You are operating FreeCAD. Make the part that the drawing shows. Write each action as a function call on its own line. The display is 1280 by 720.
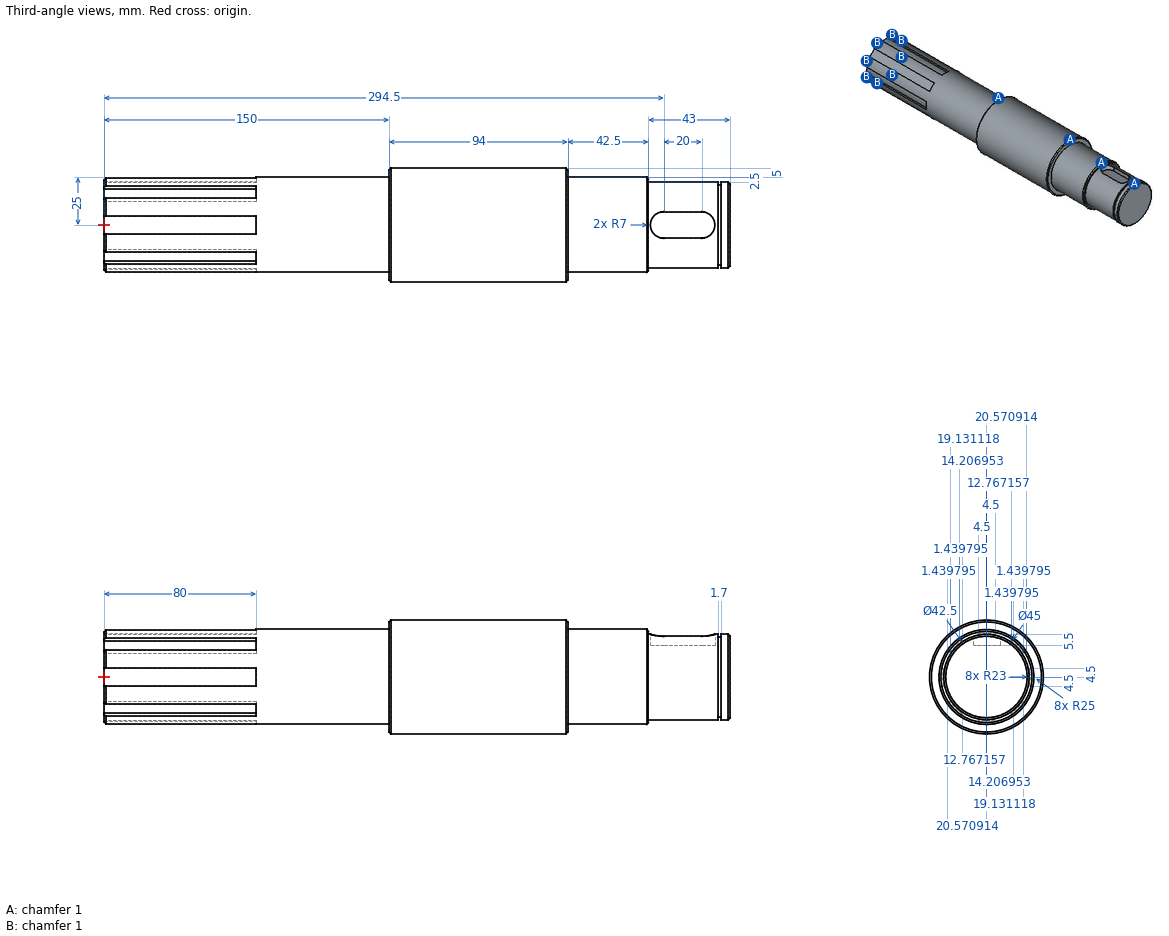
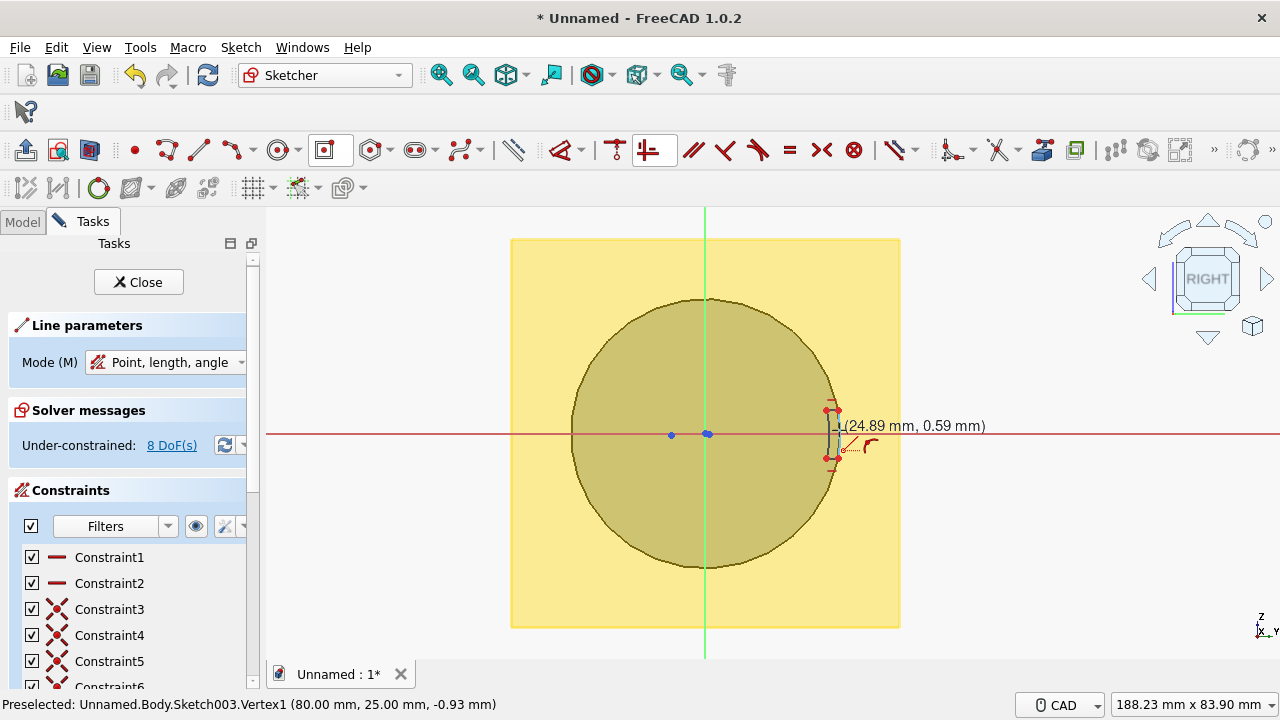
click(774, 331)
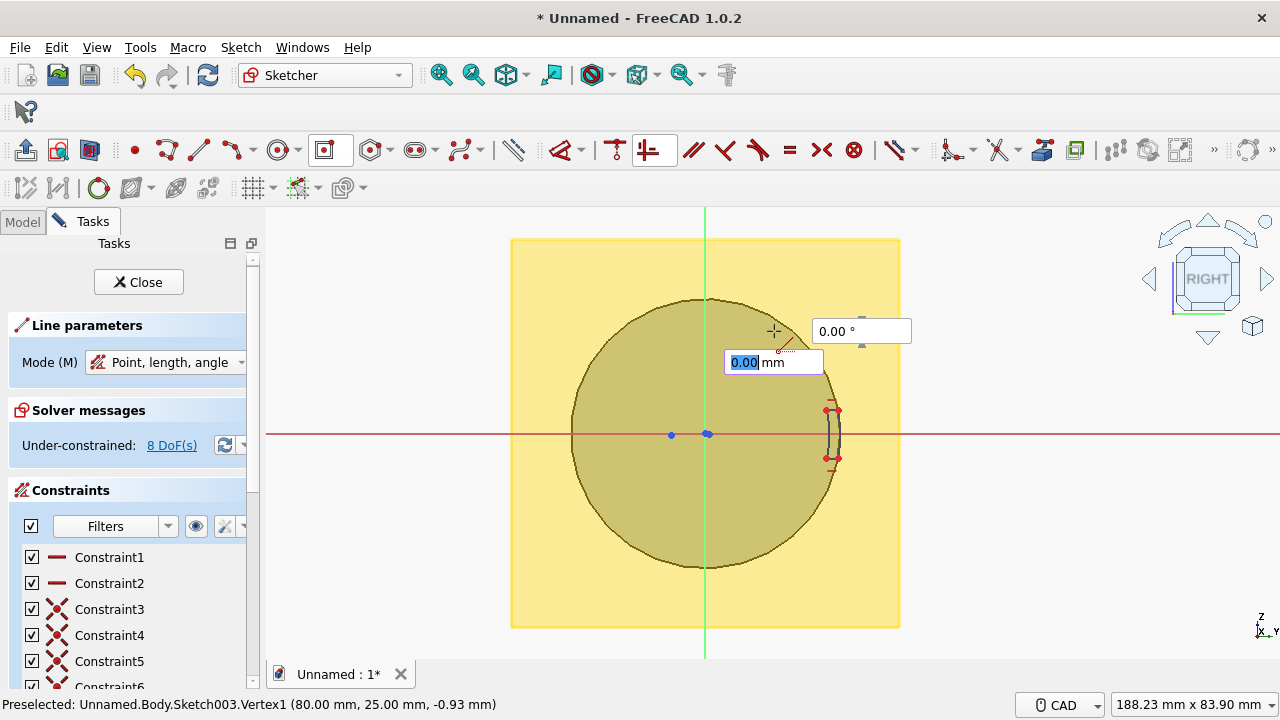
scroll(782, 323, up, 2)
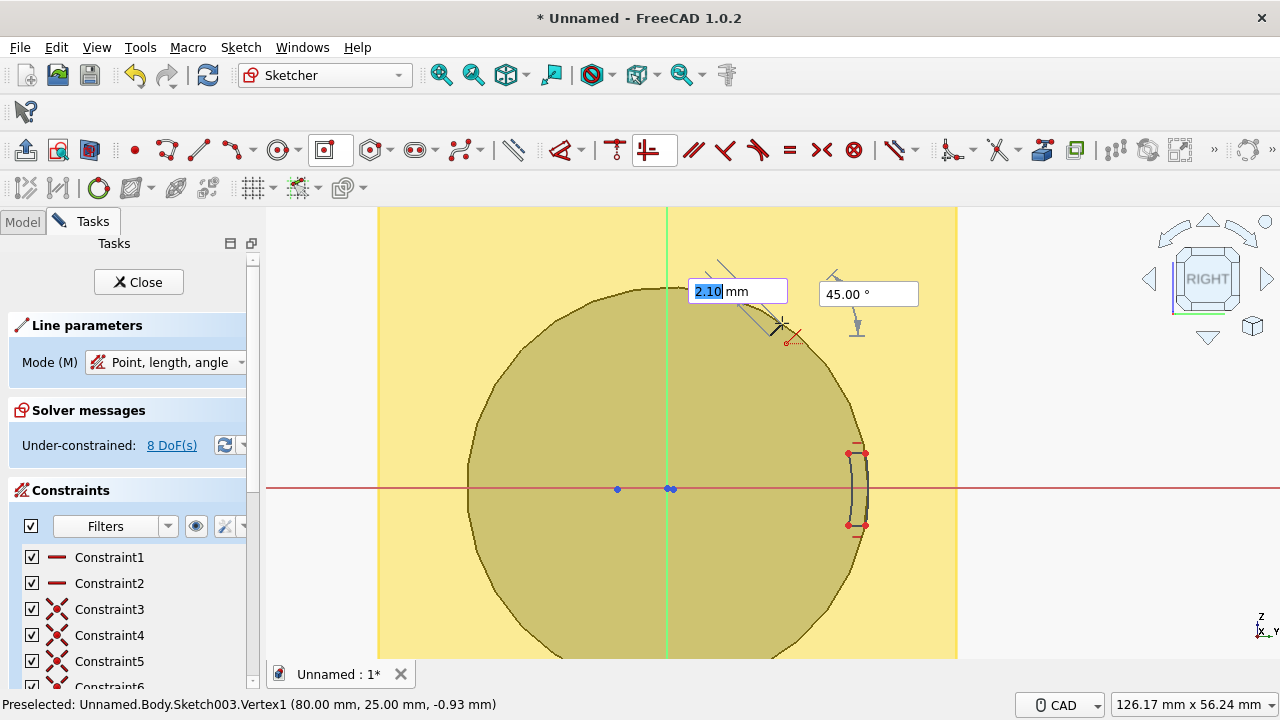
click(782, 323)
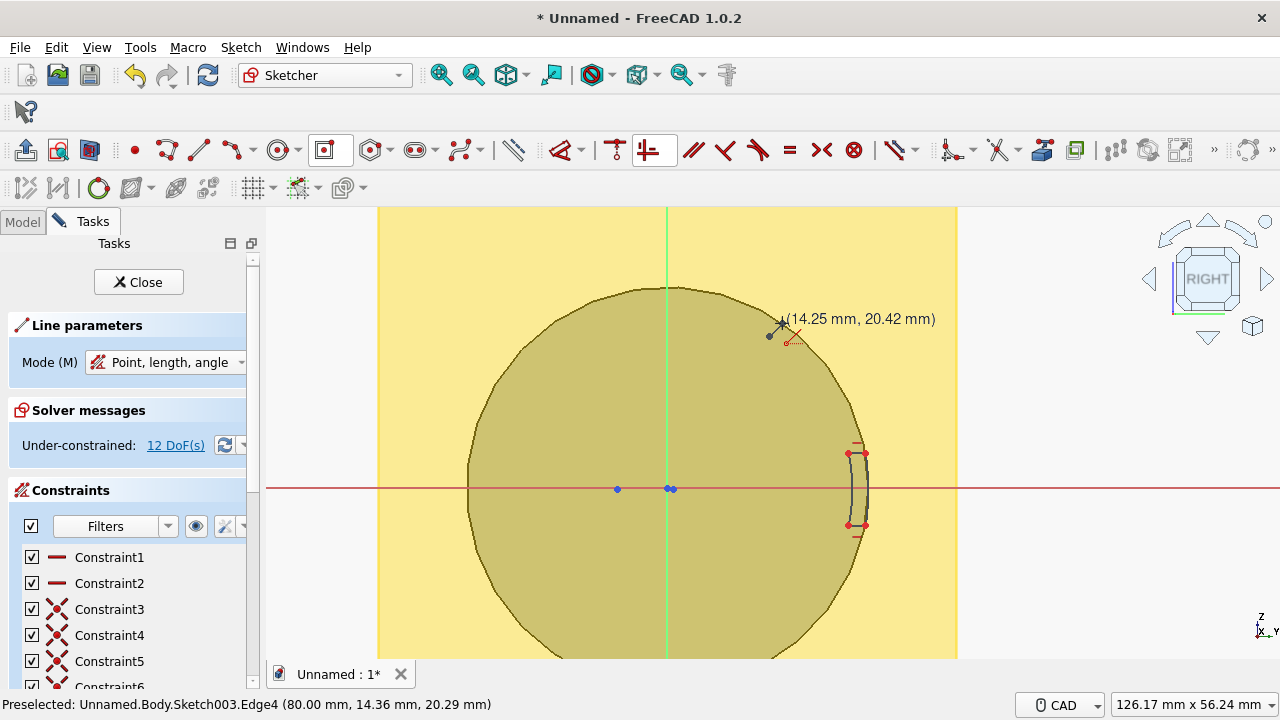
click(833, 374)
click(821, 385)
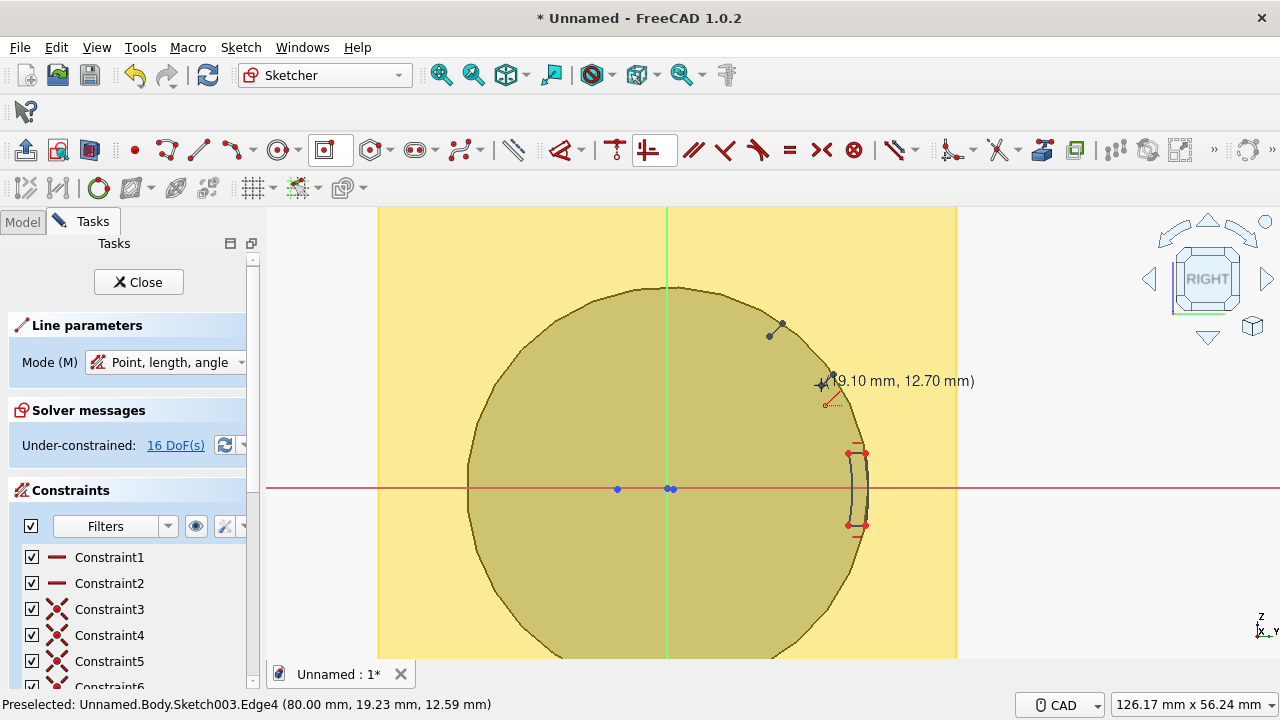
click(232, 150)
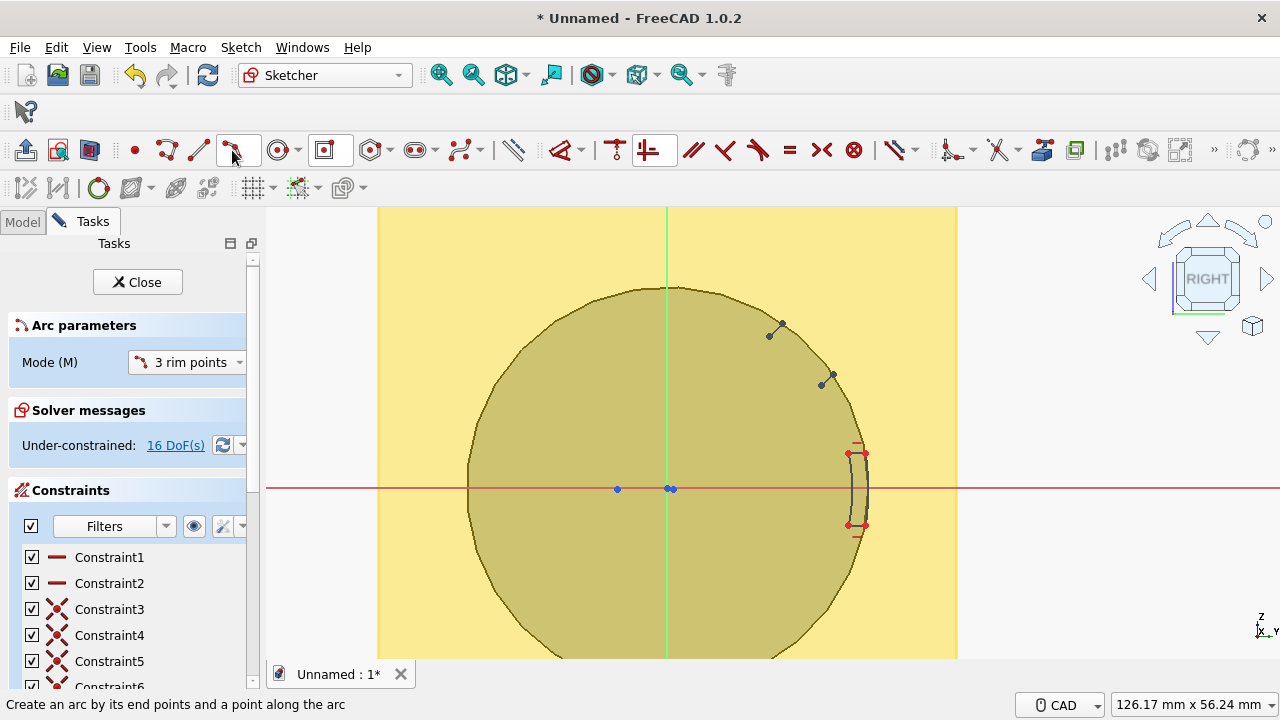
scroll(782, 323, up, 4)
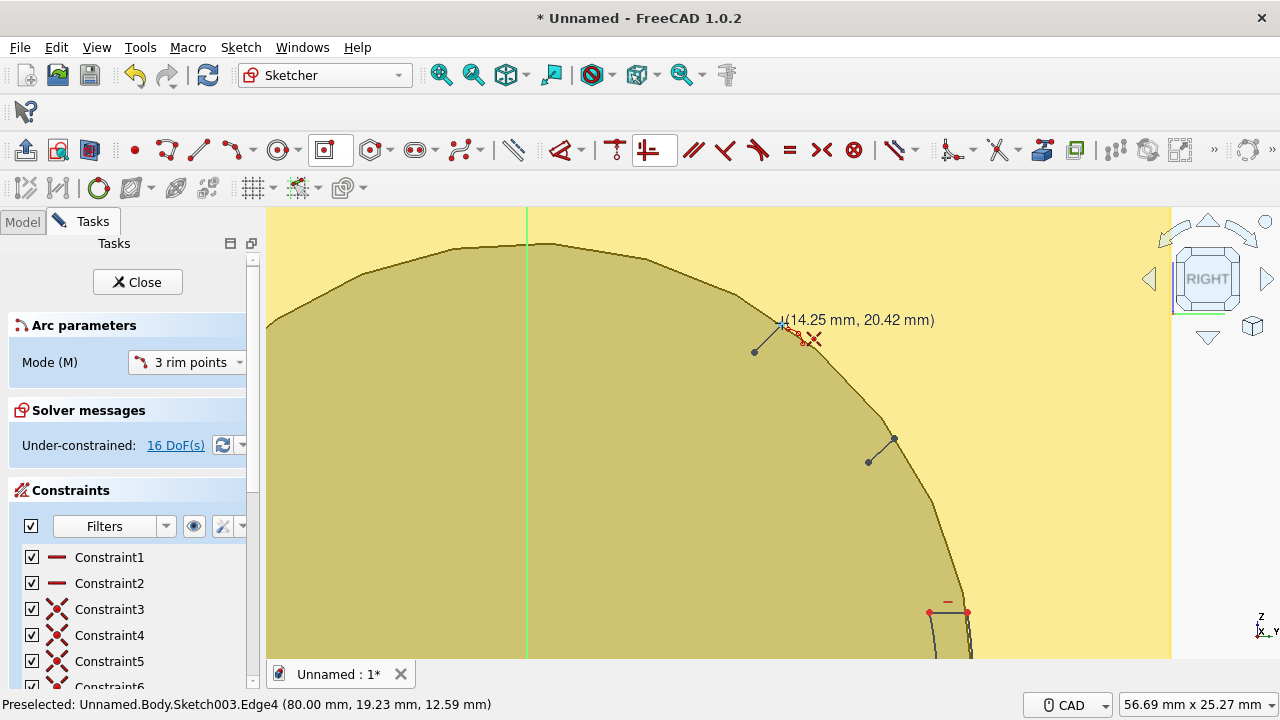
click(781, 325)
click(895, 438)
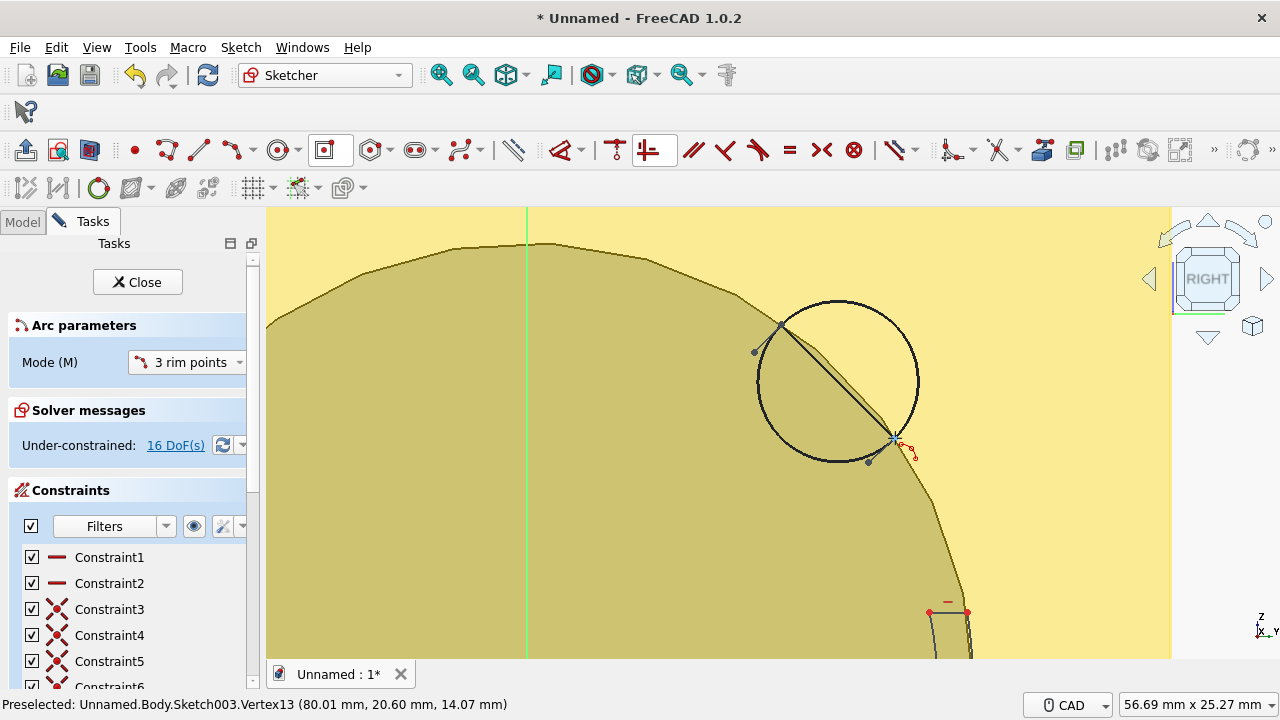
scroll(843, 374, up, 4)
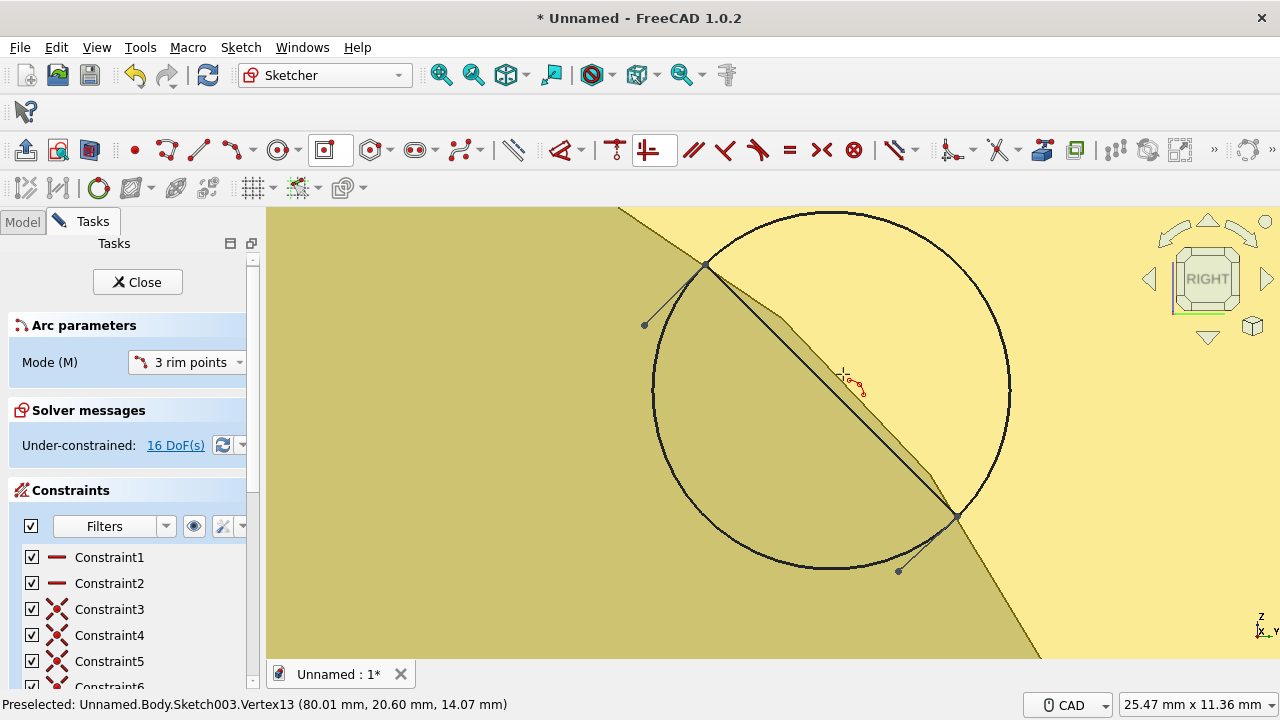
click(842, 373)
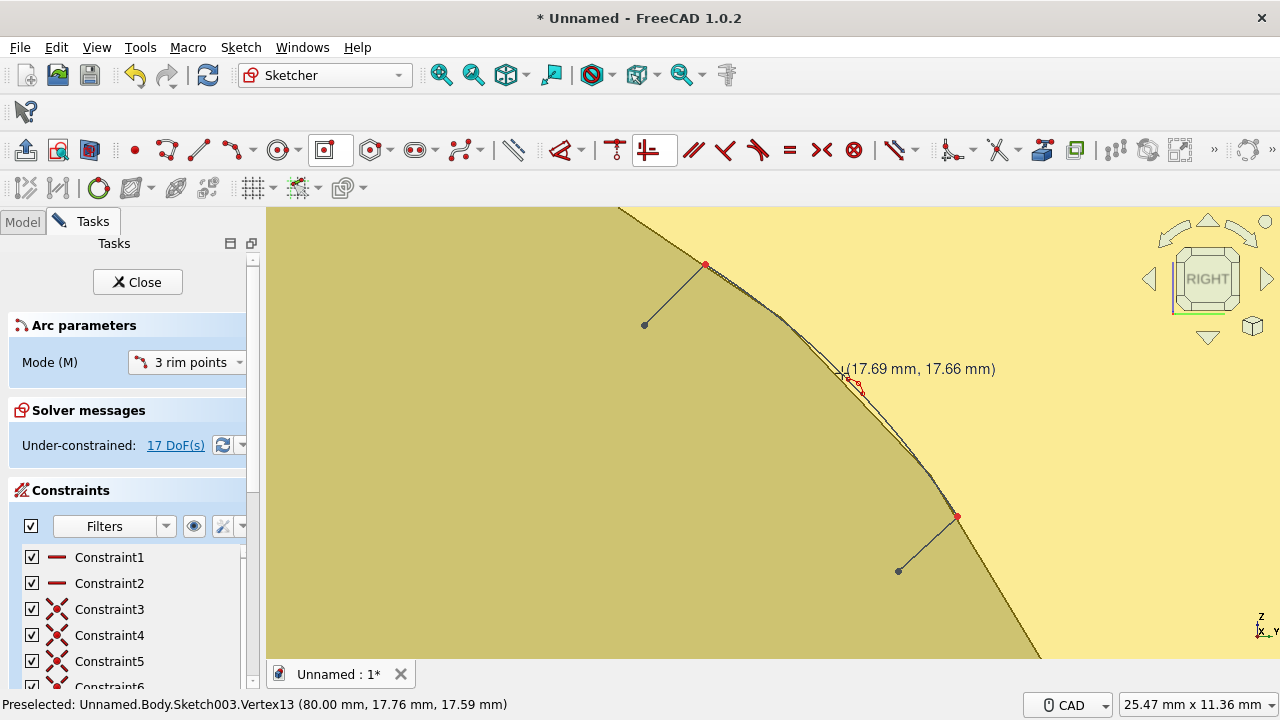
click(898, 571)
click(645, 325)
click(785, 430)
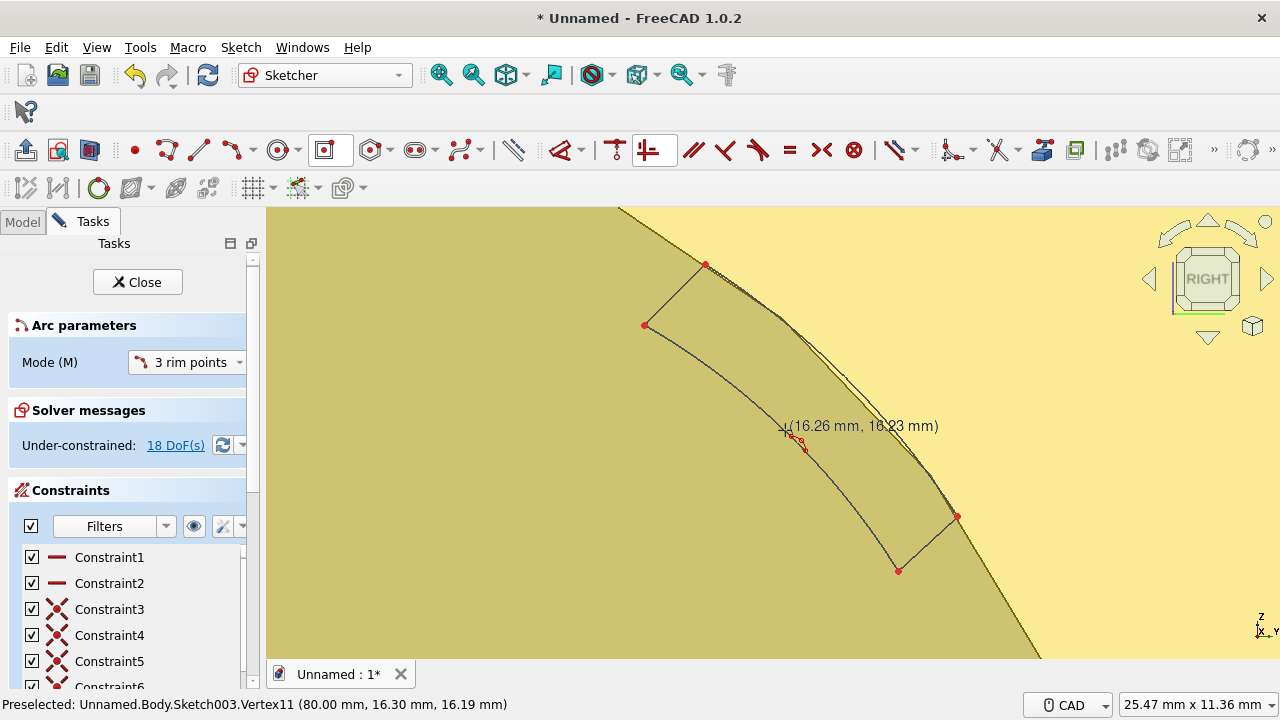
click(200, 150)